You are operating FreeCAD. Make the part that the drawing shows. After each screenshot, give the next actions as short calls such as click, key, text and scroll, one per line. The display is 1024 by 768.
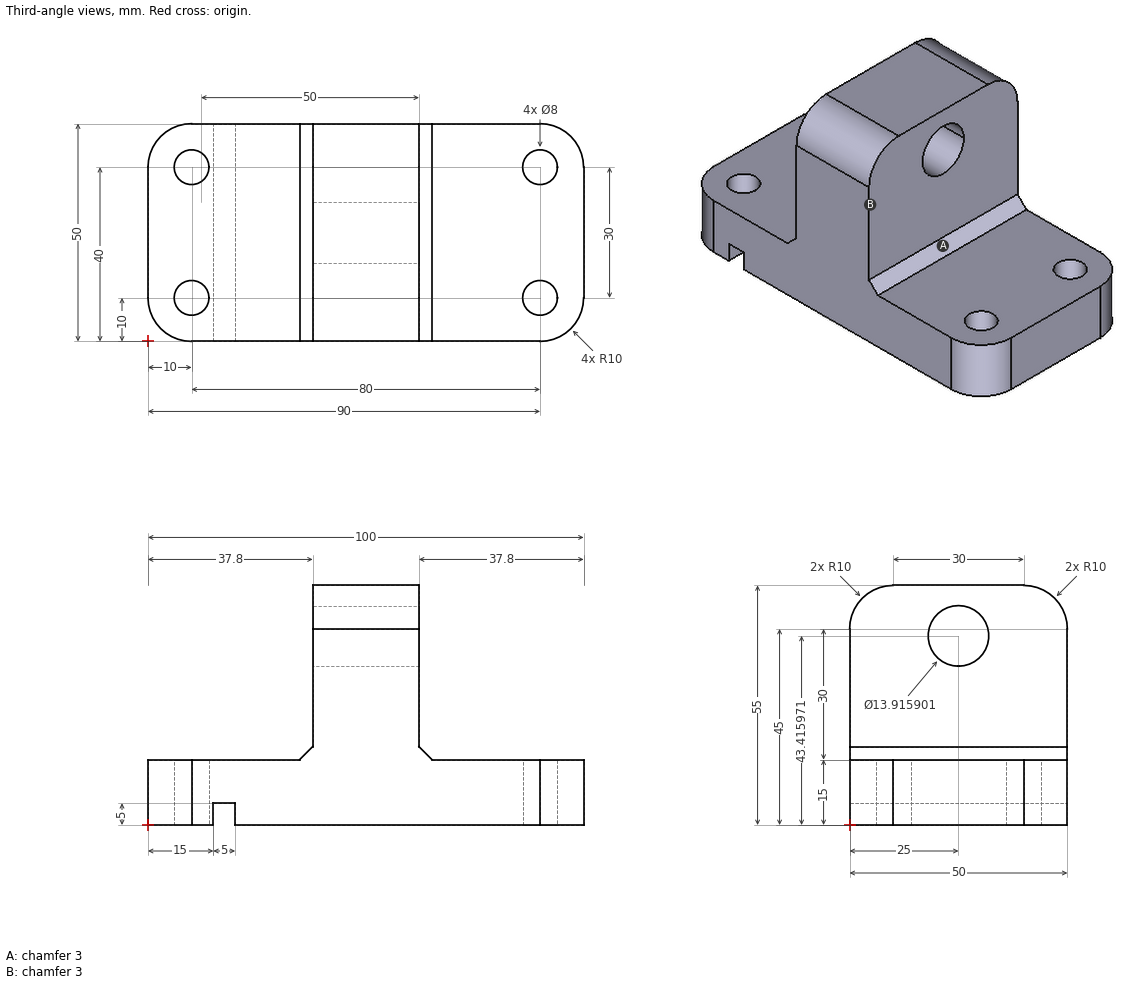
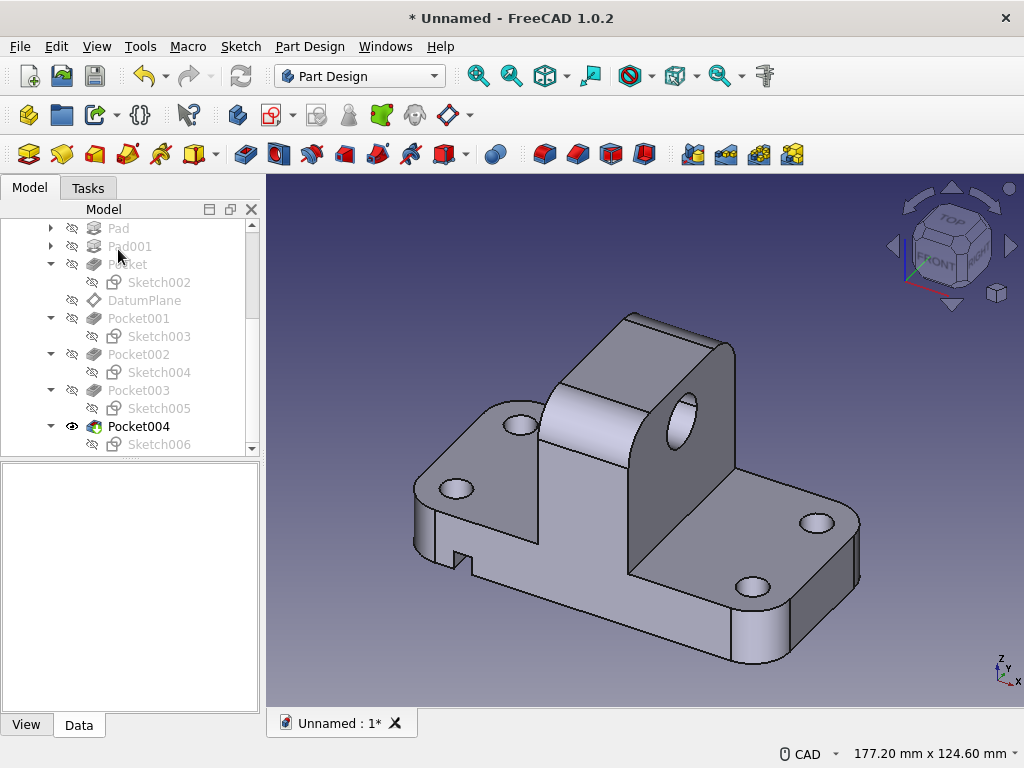
key(0)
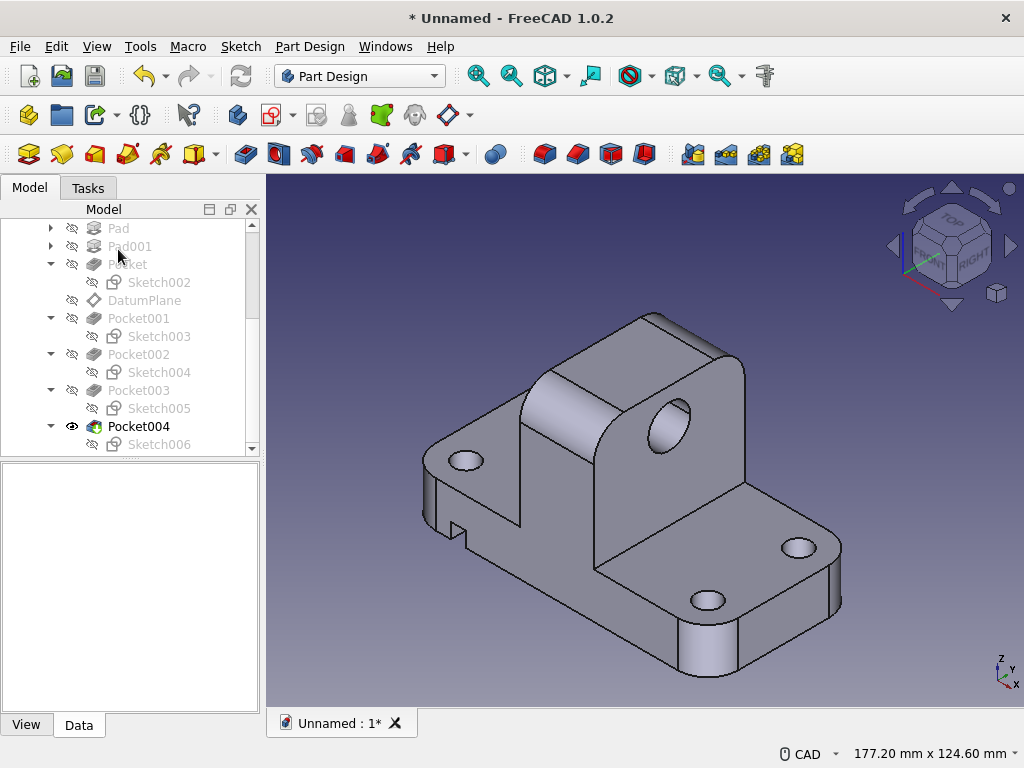
key(2)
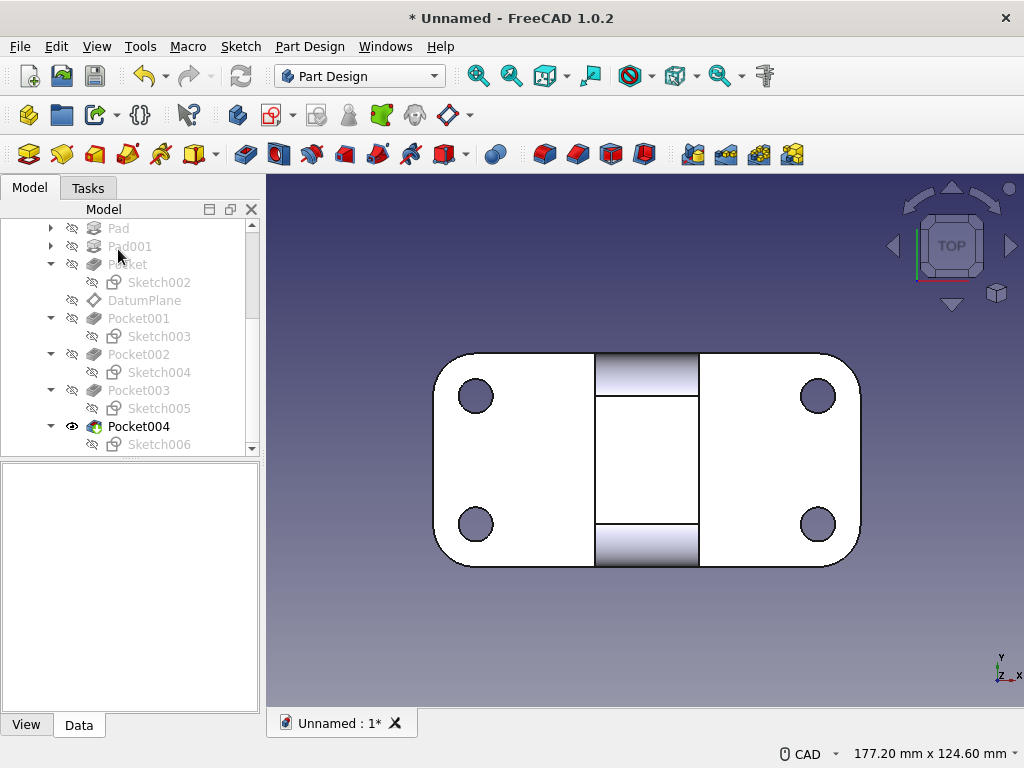
key(1)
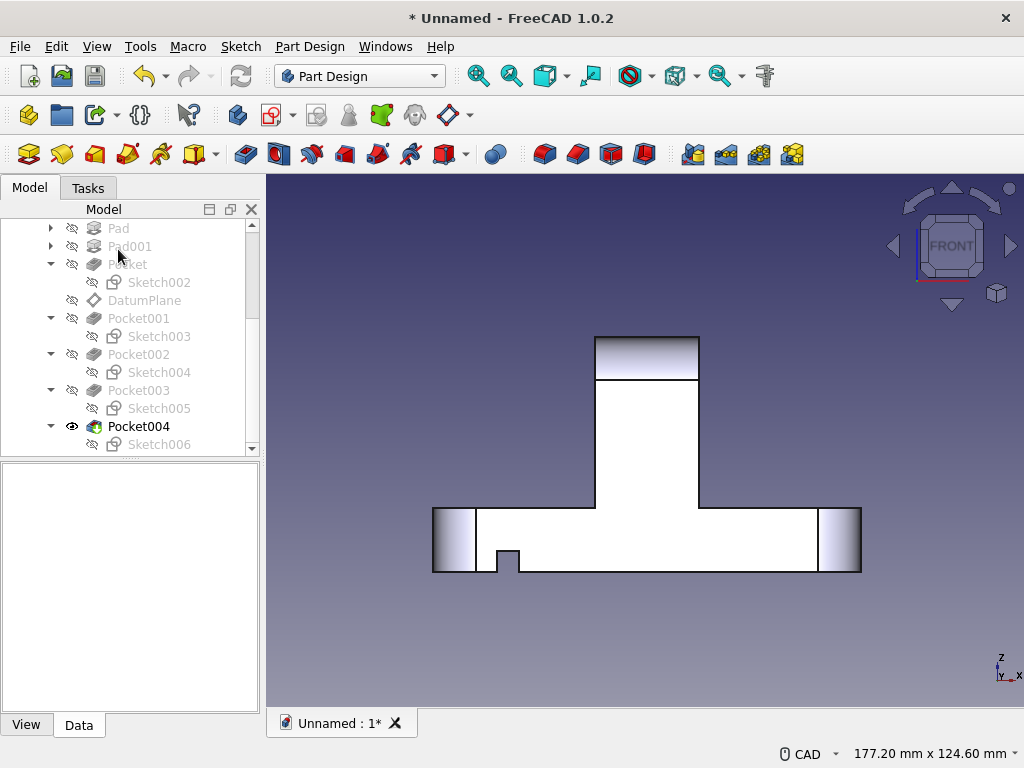
key(3)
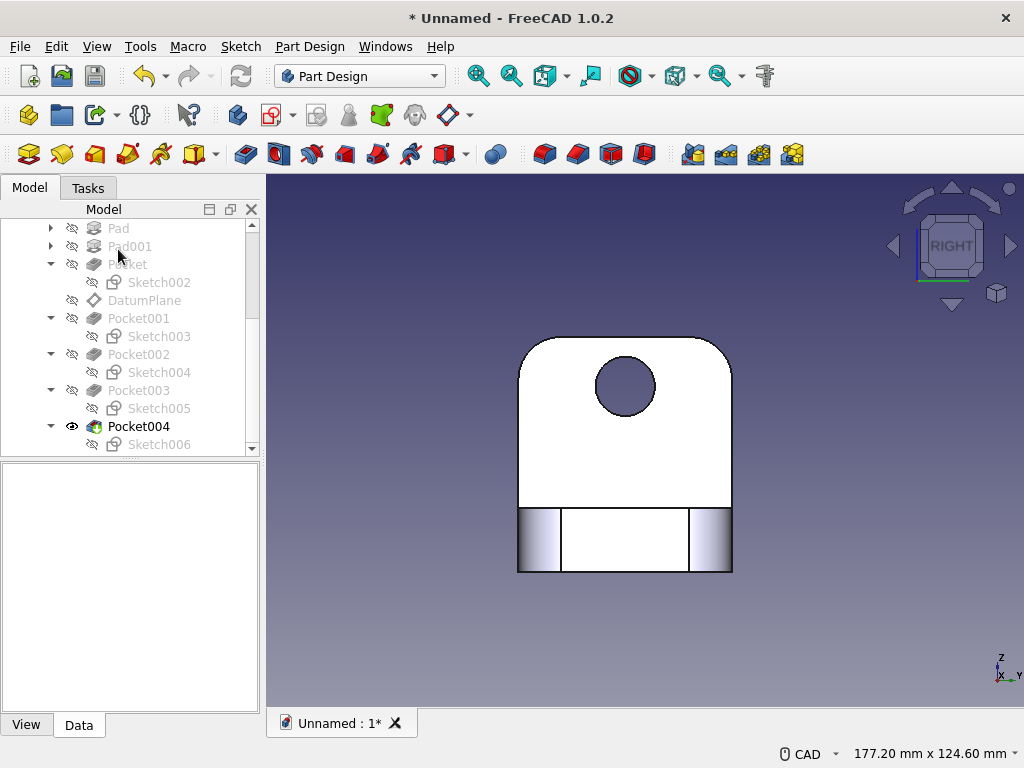
click(479, 76)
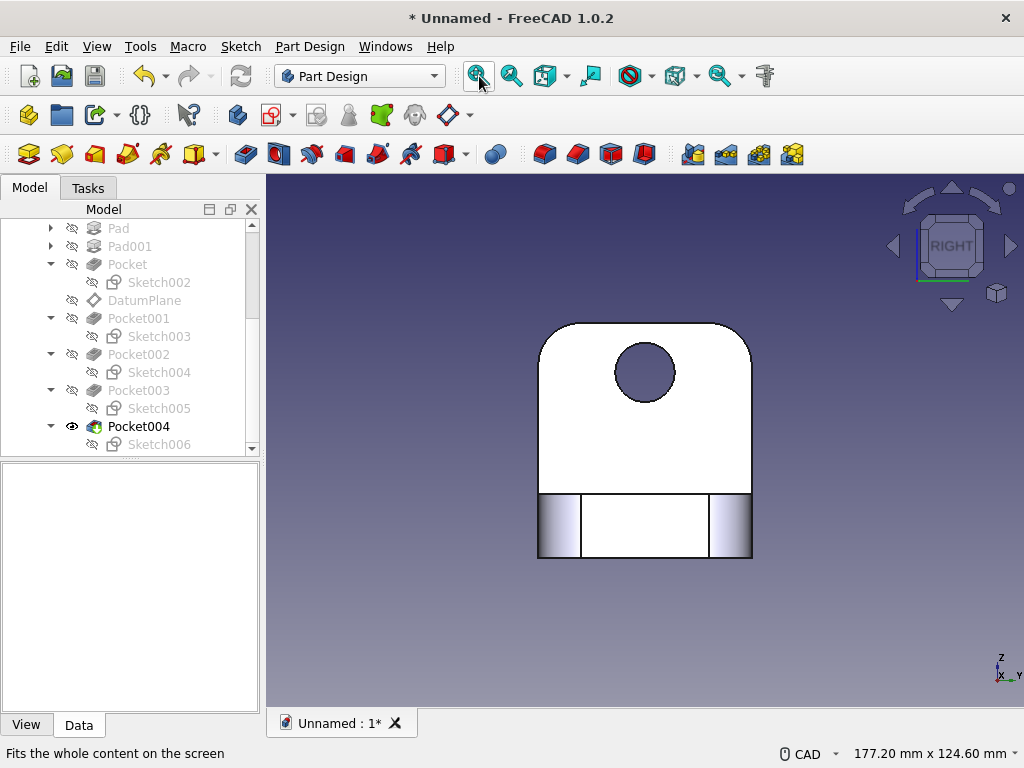
key(5)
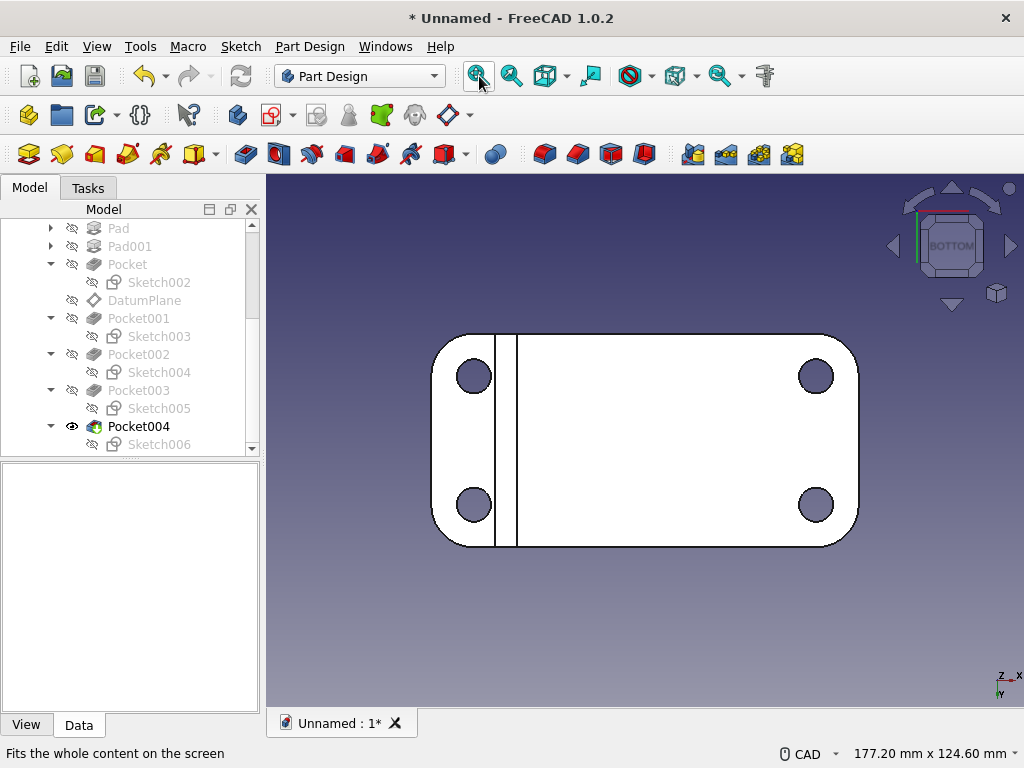
key(4)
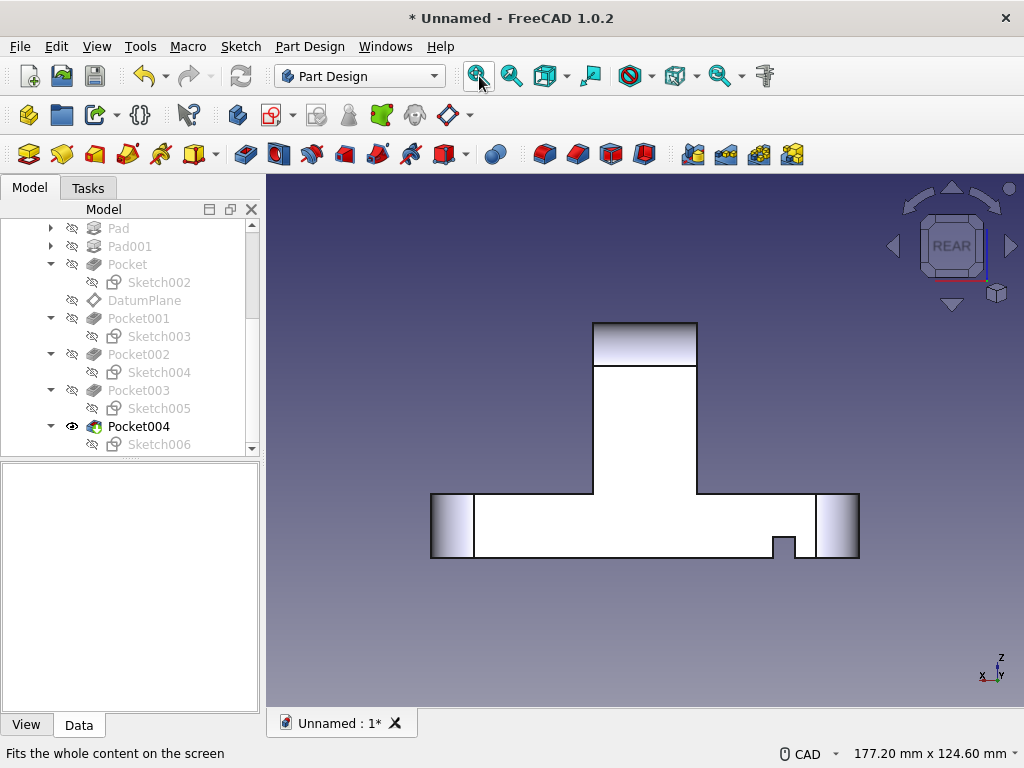
key(6)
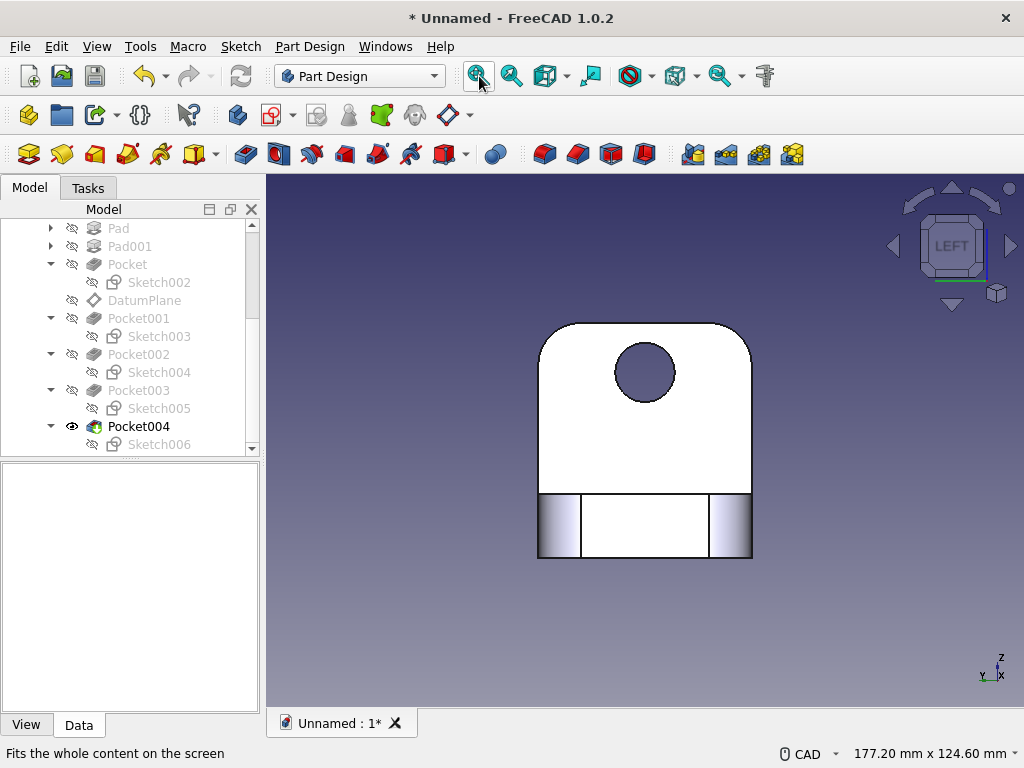
click(479, 76)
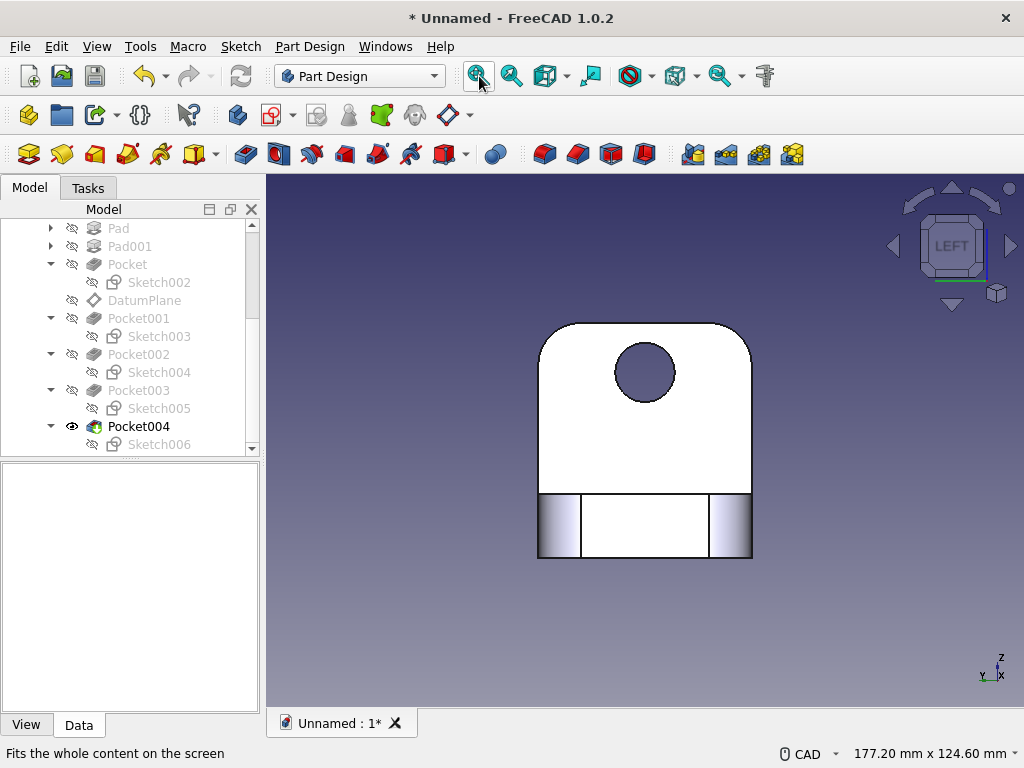
key(v)
key(3)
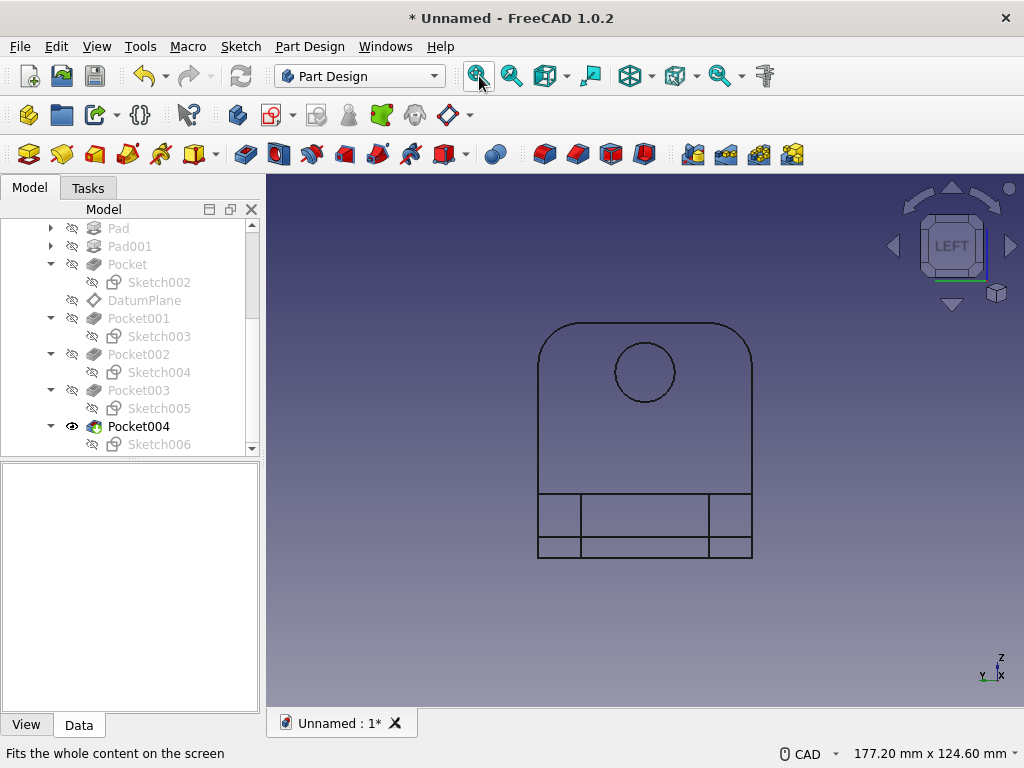
key(0)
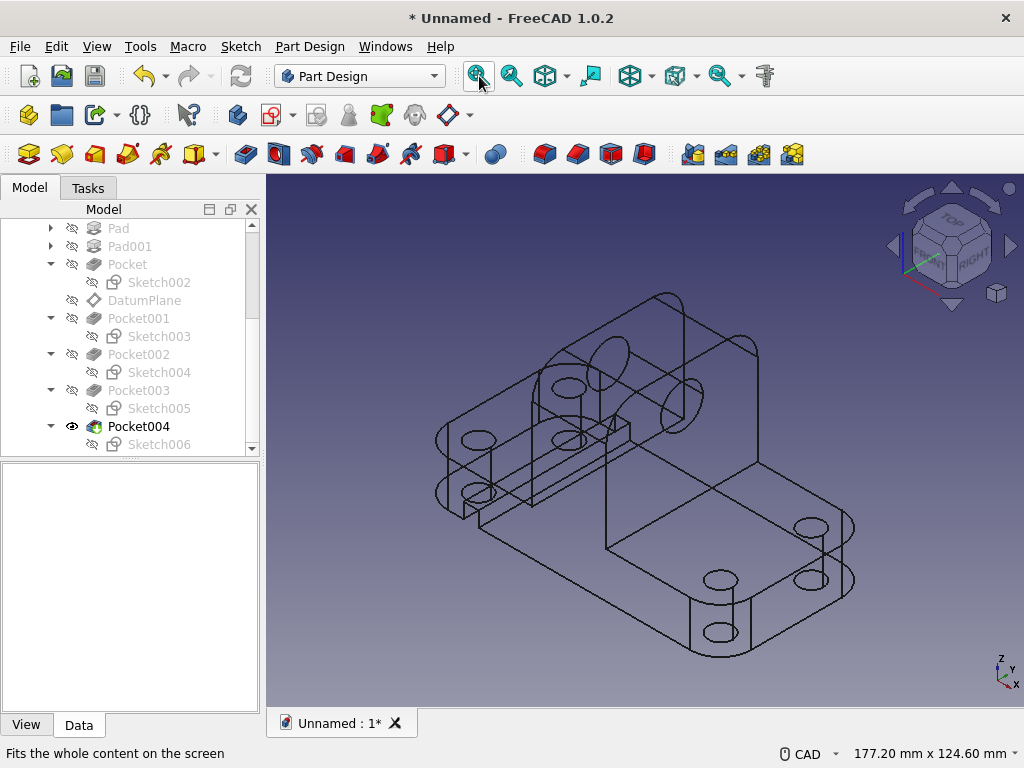
click(682, 504)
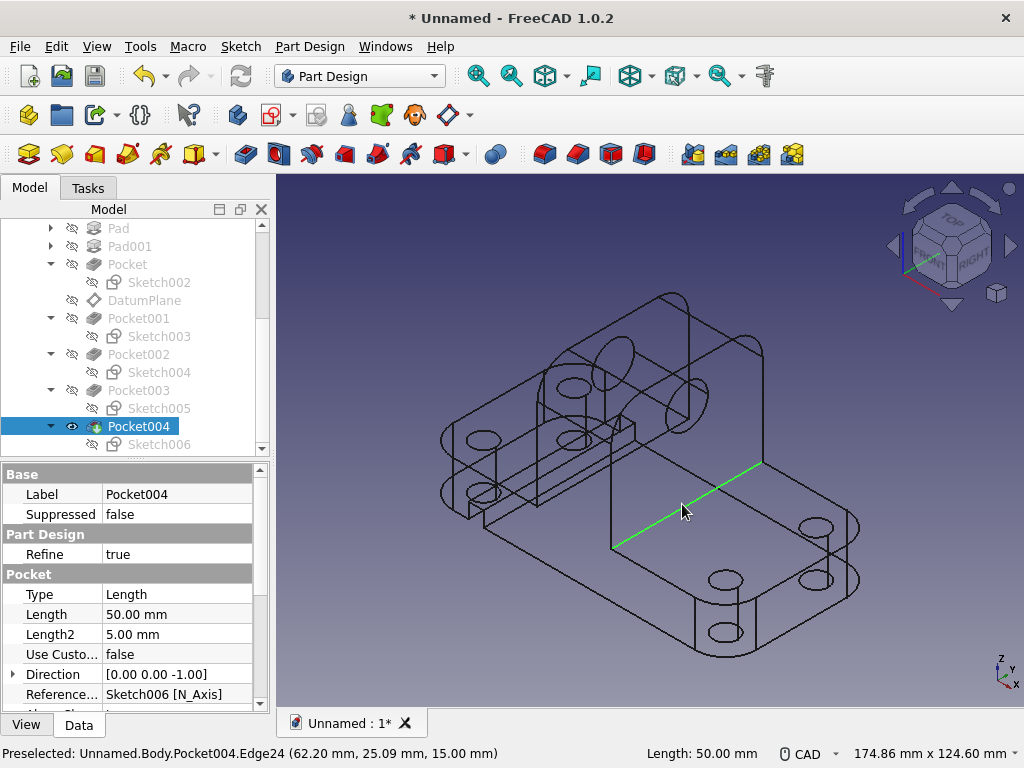
key(v)
key(1)